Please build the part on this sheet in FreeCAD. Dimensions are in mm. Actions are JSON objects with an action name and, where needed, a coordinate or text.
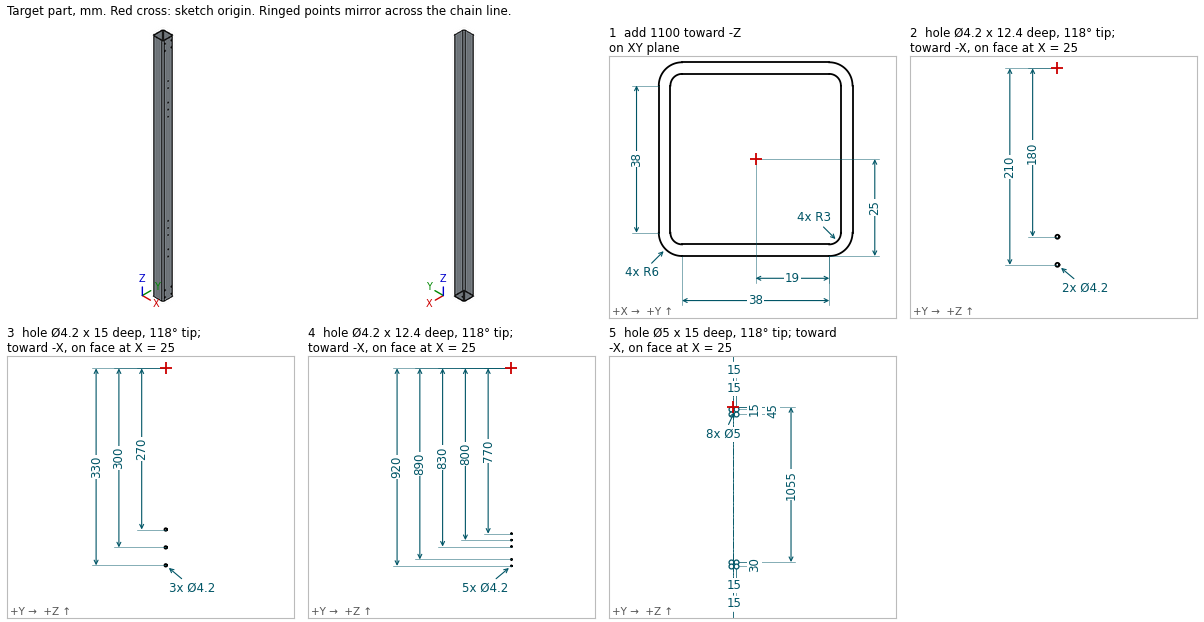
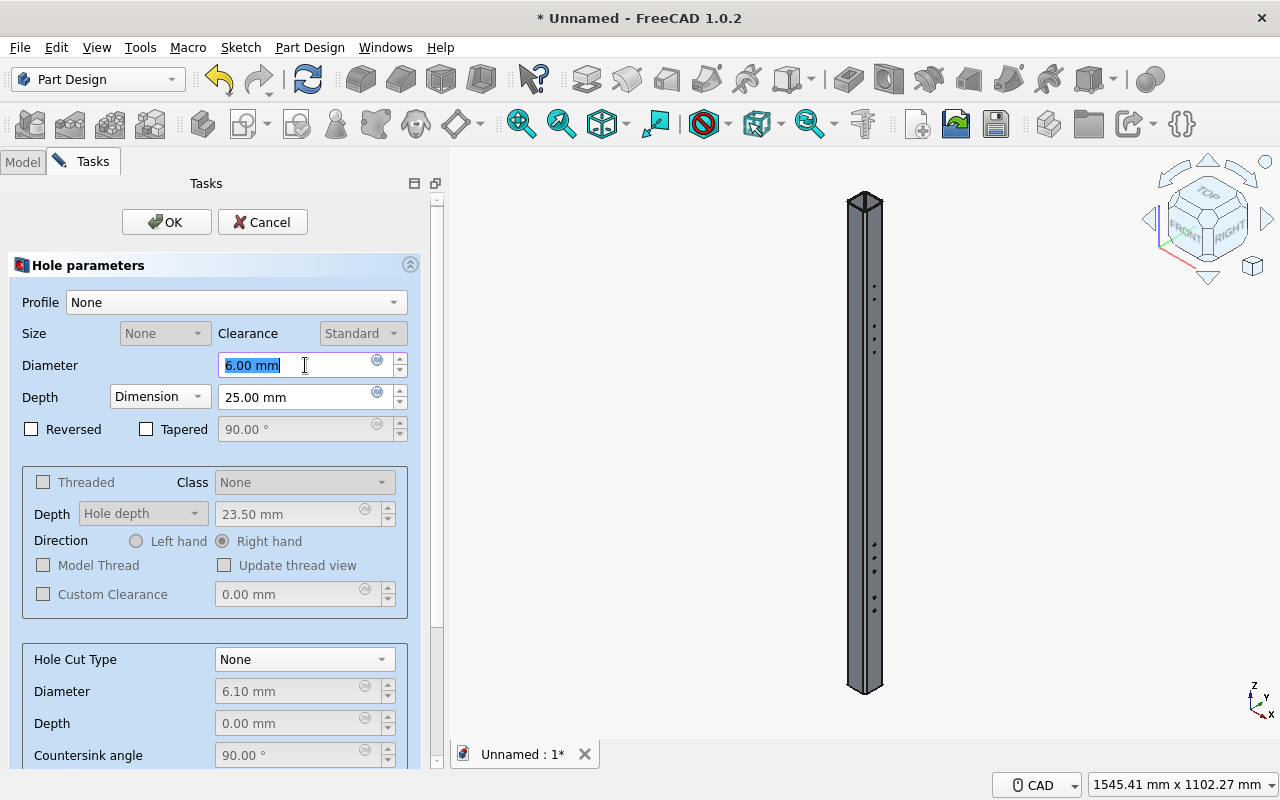
{"action": "type", "text": "4.2"}
{"action": "key", "text": "Tab"}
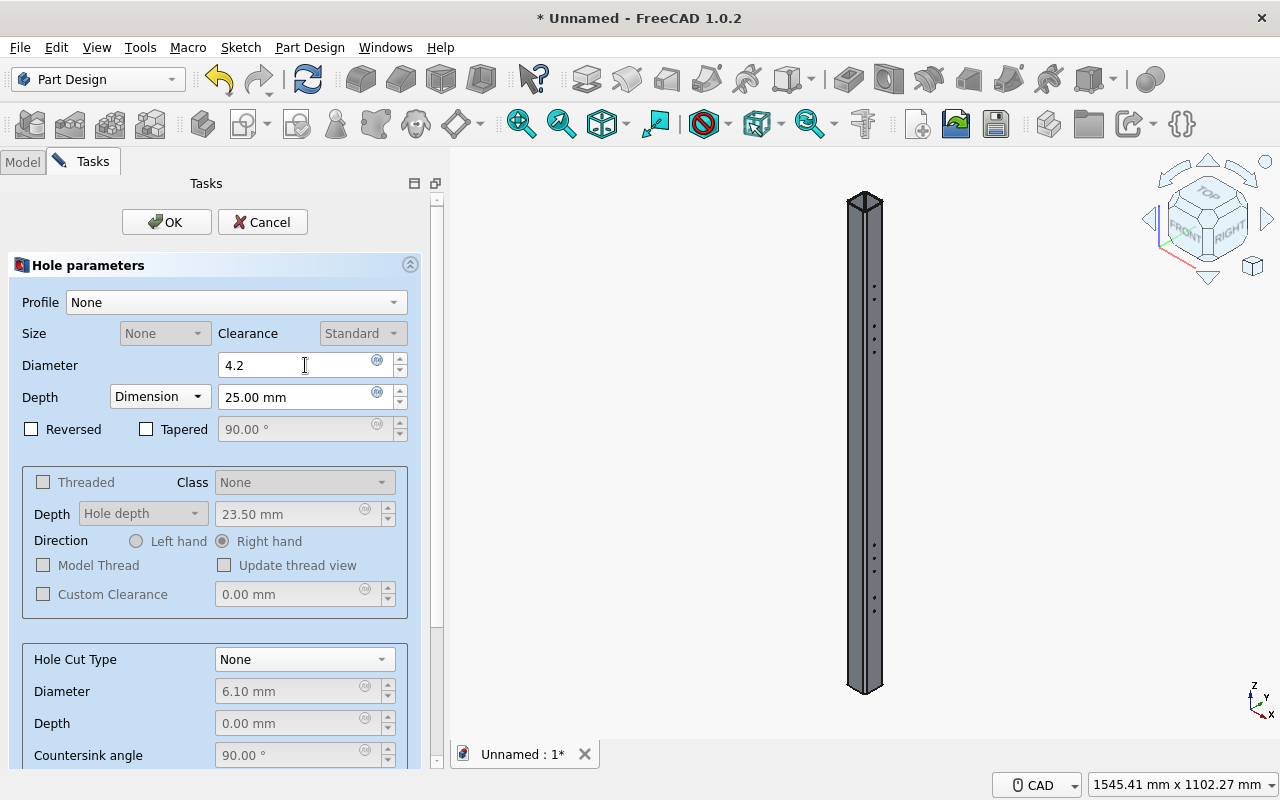
{"action": "triple_click", "coordinate": [305, 397]}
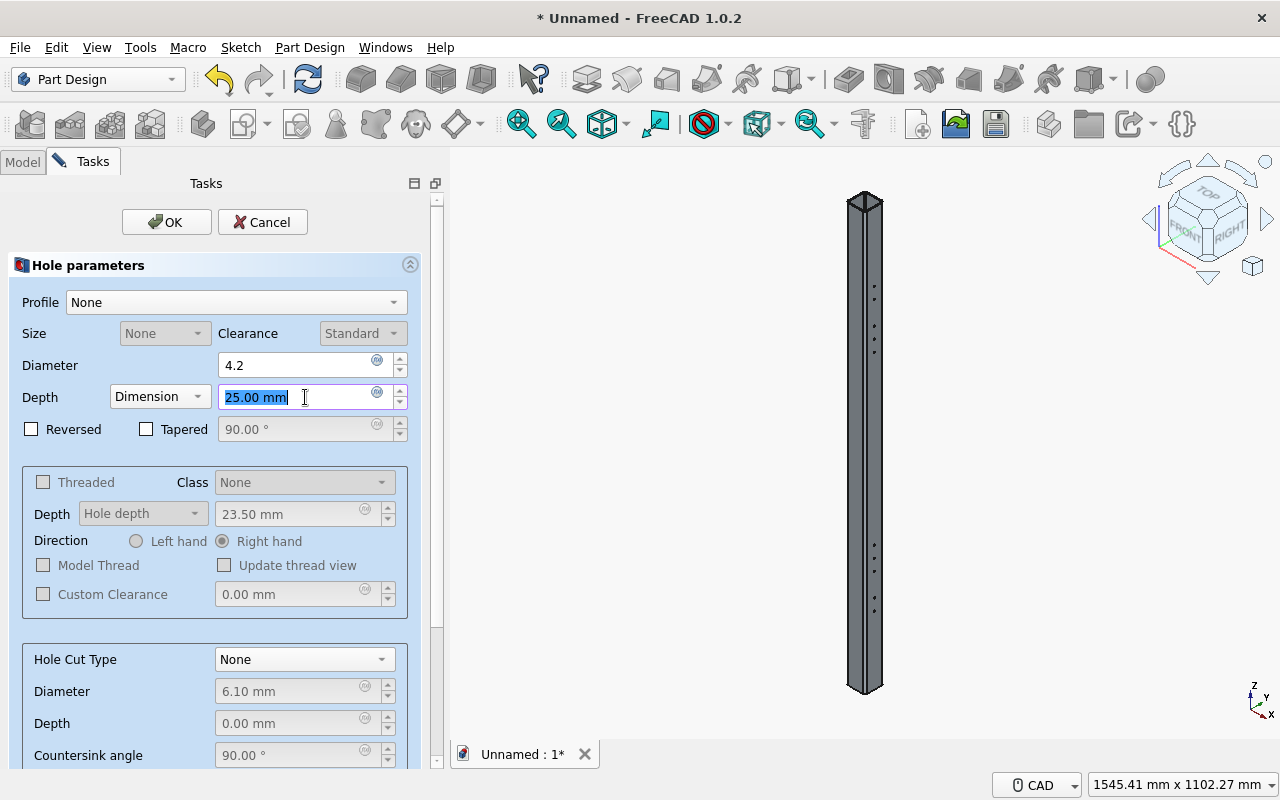
{"action": "type", "text": "12.4"}
{"action": "key", "text": "Tab"}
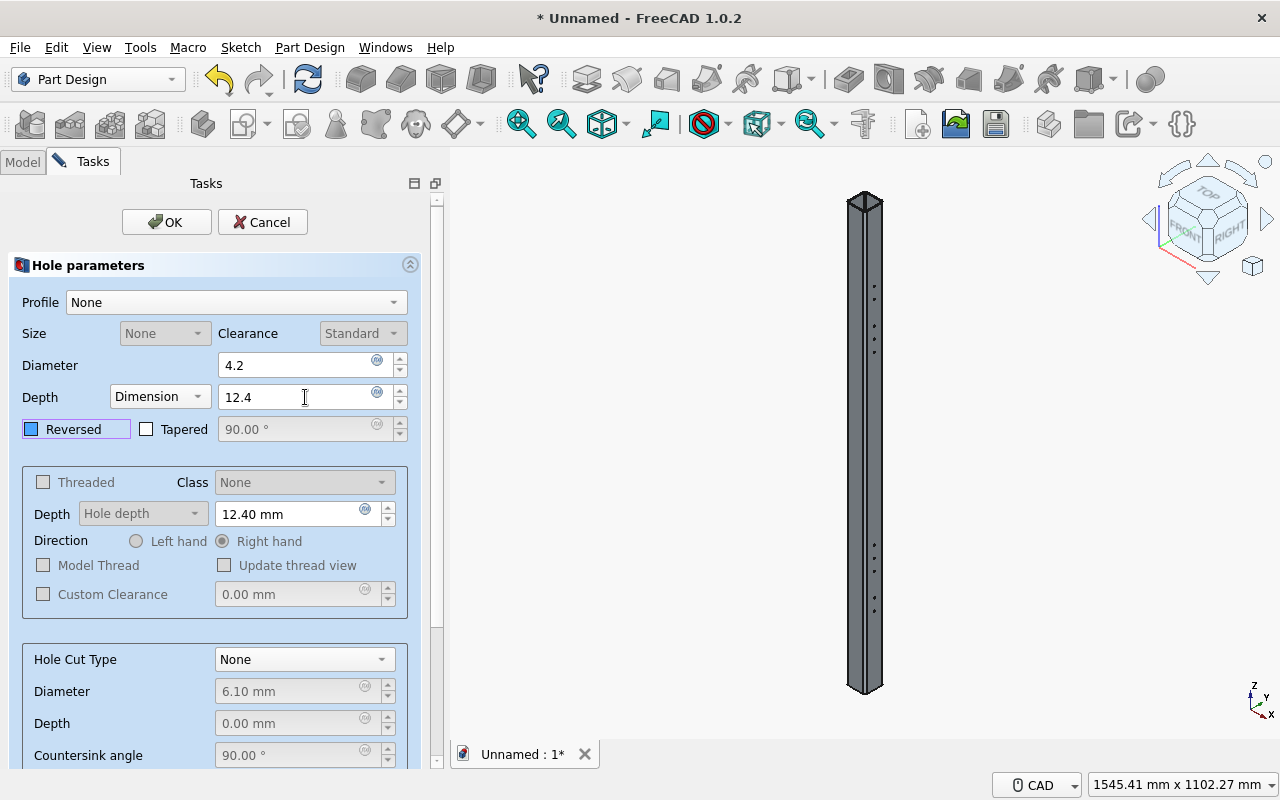
{"action": "left_click", "coordinate": [167, 222]}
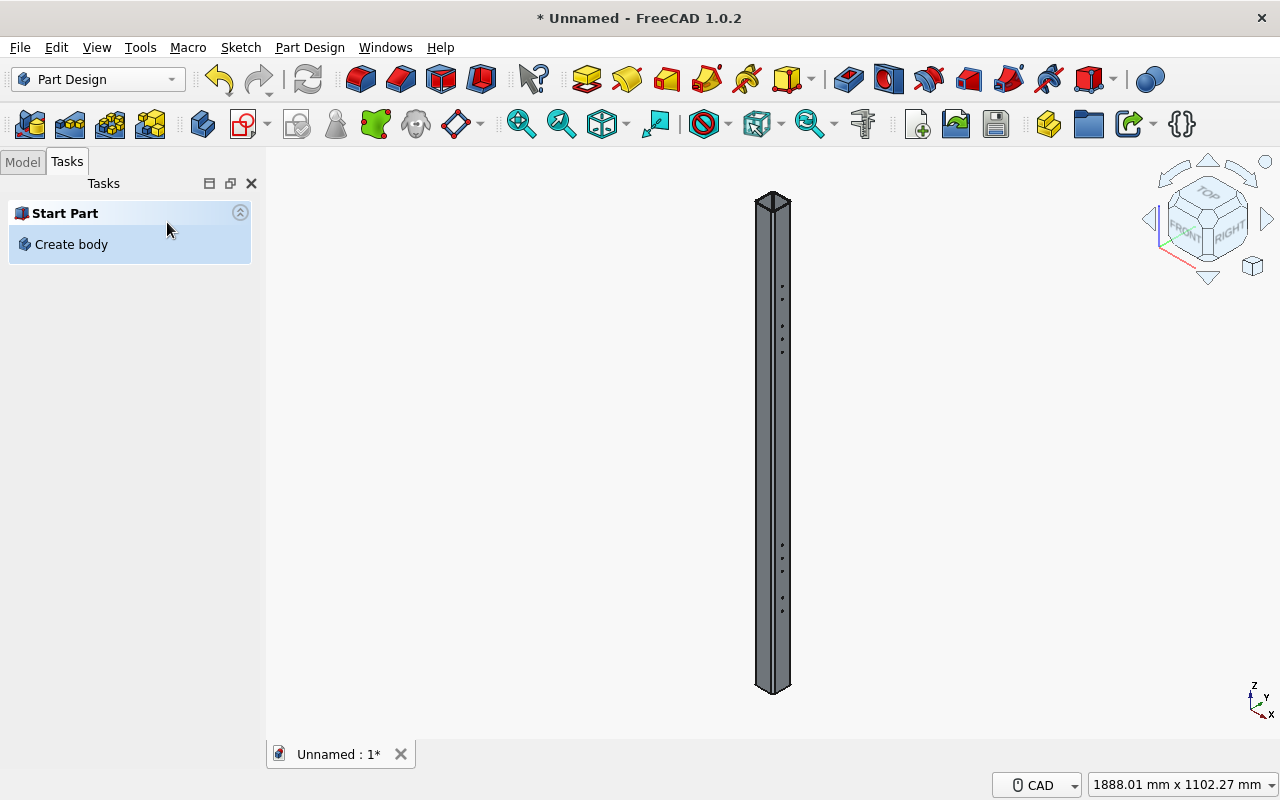
{"action": "left_click", "coordinate": [785, 240]}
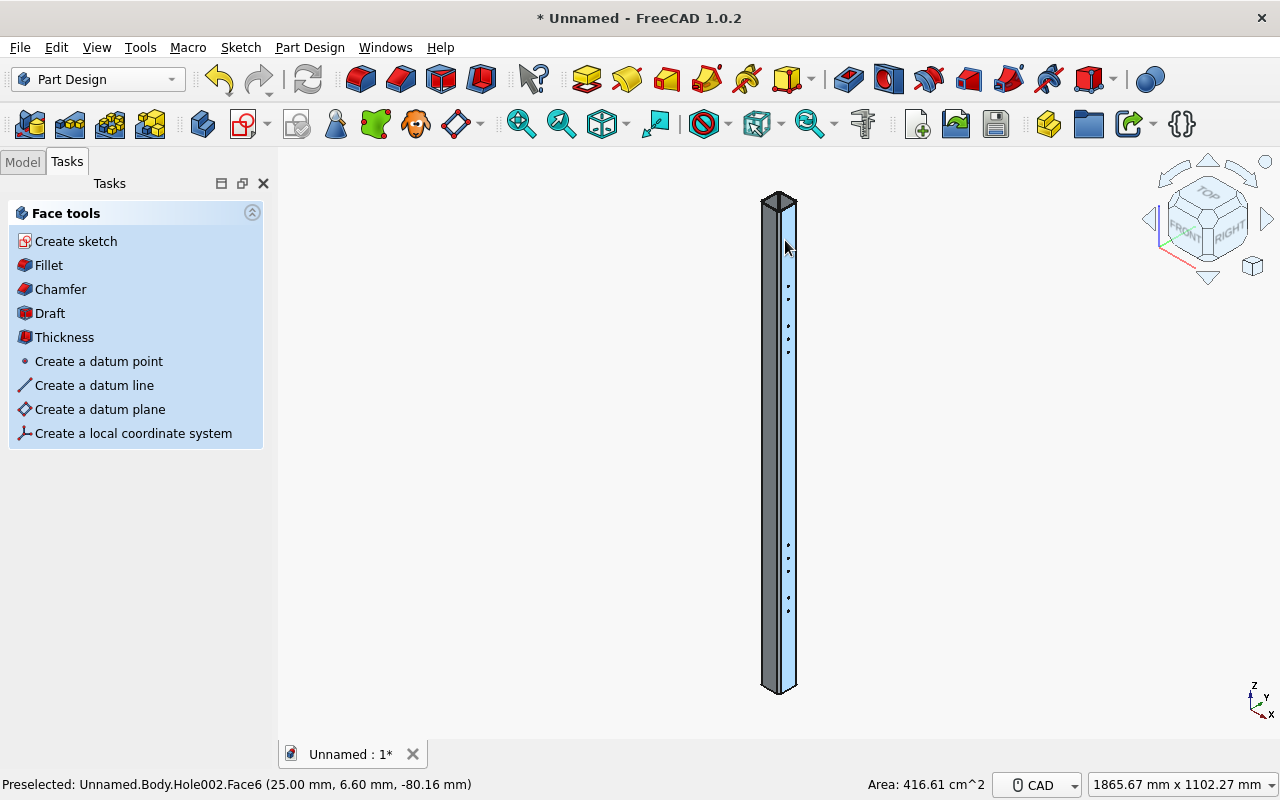
{"action": "left_click", "coordinate": [244, 124]}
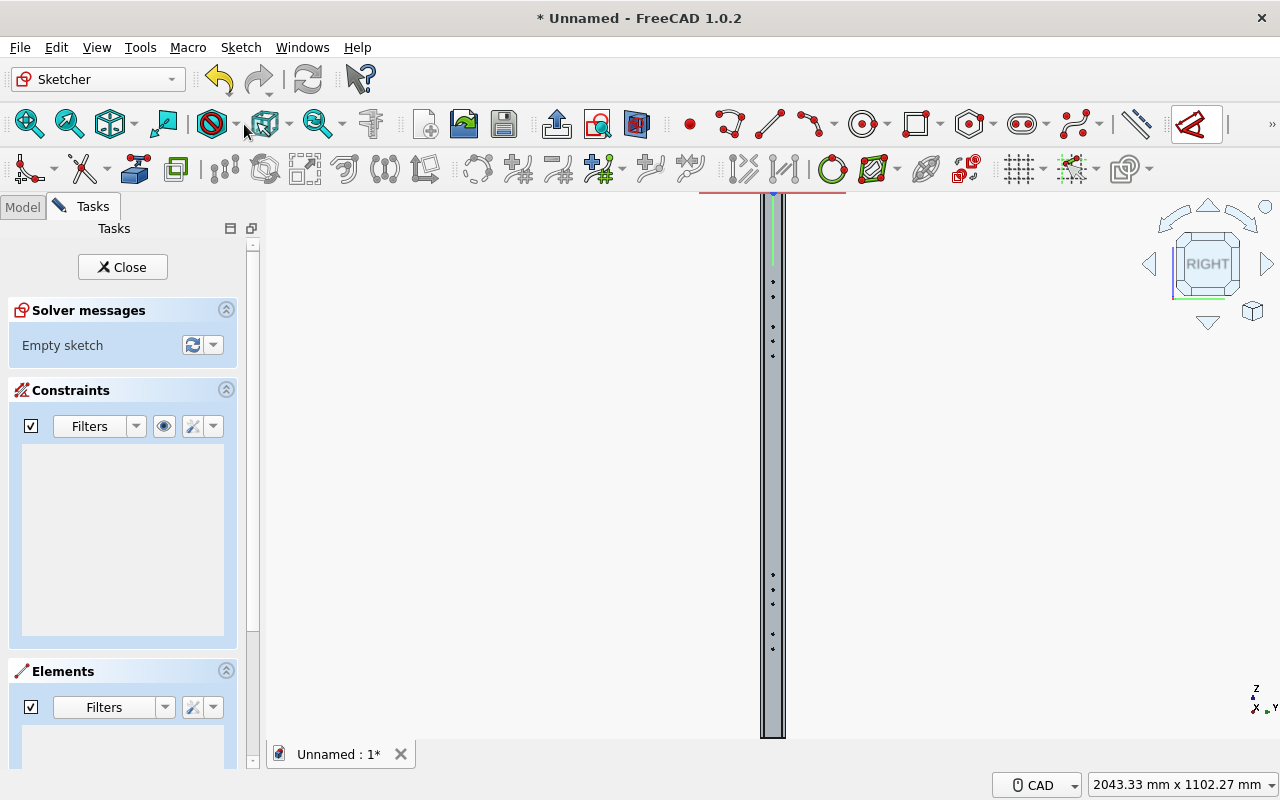
{"action": "scroll", "coordinate": [565, 472], "scroll_direction": "down", "scroll_amount": 2}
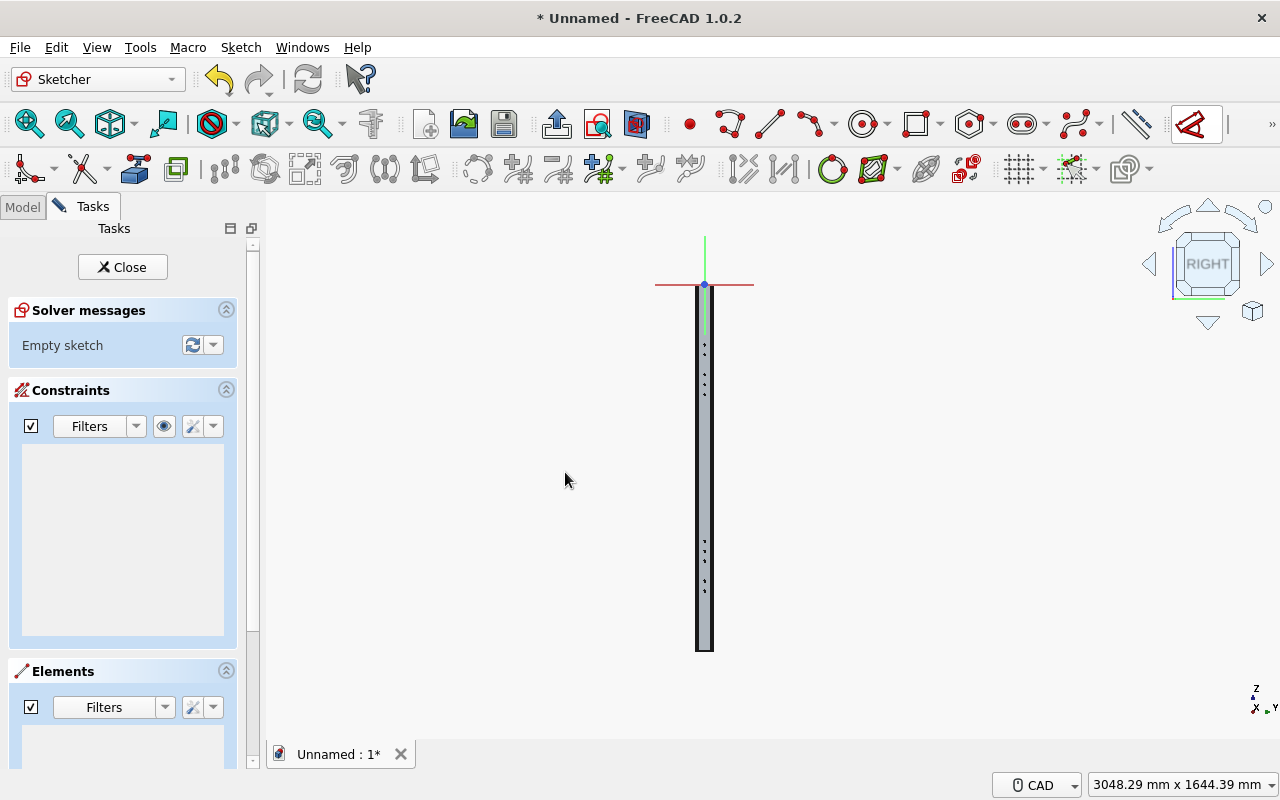
{"action": "left_click", "coordinate": [864, 124]}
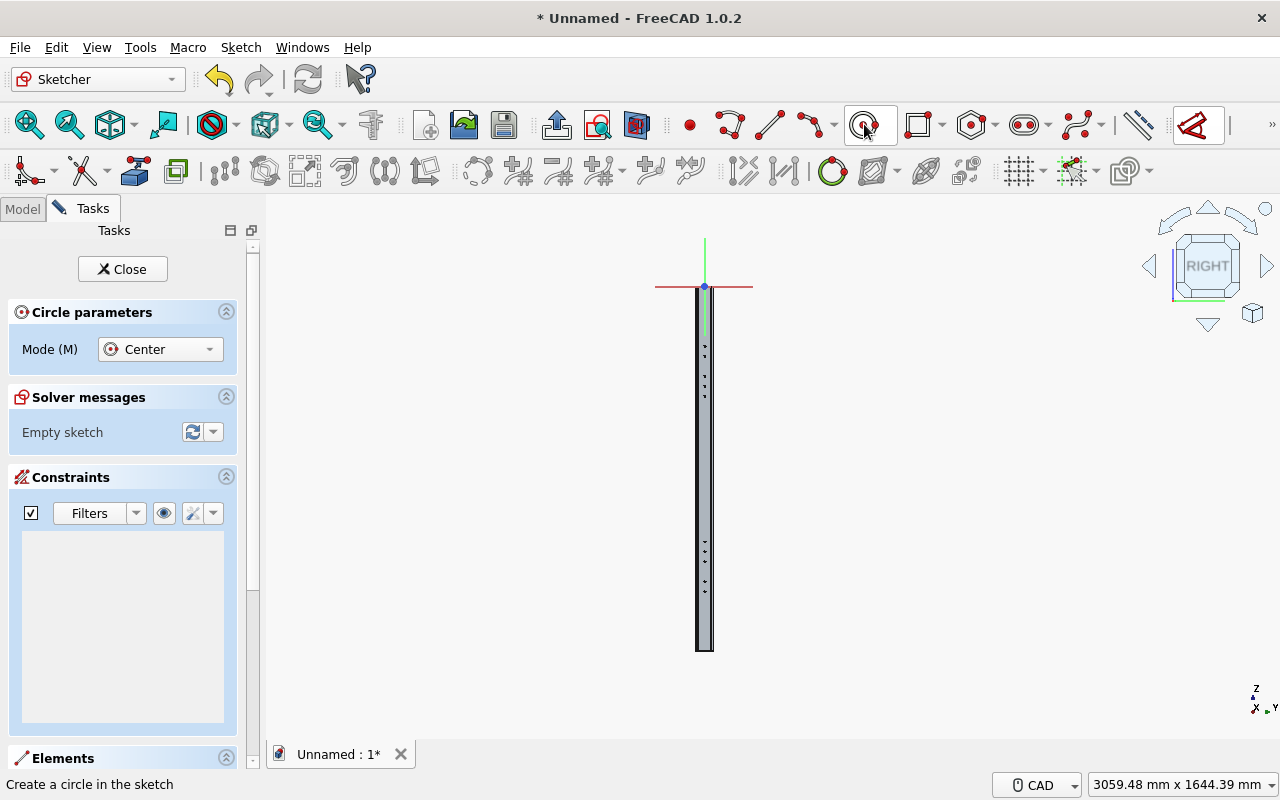
{"action": "scroll", "coordinate": [710, 291], "scroll_direction": "up", "scroll_amount": 17}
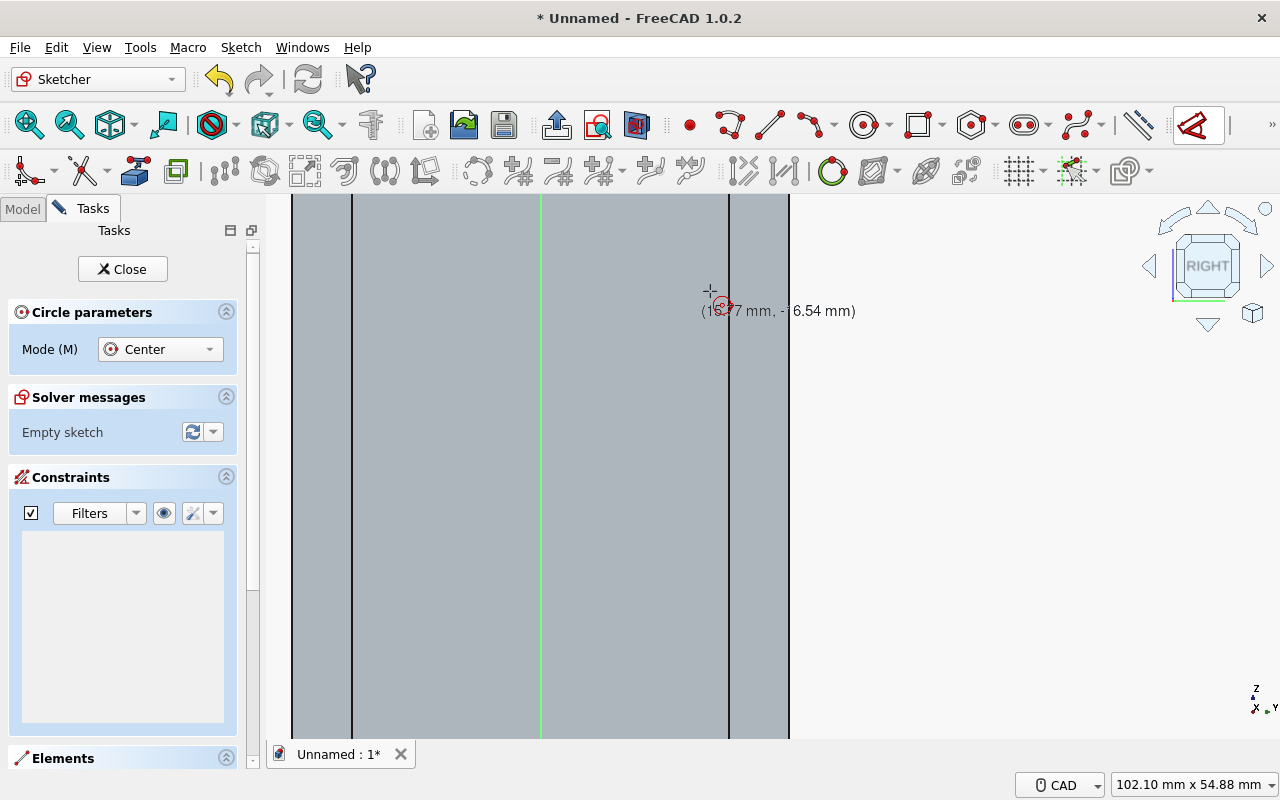
{"action": "scroll", "coordinate": [710, 291], "scroll_direction": "down", "scroll_amount": 17}